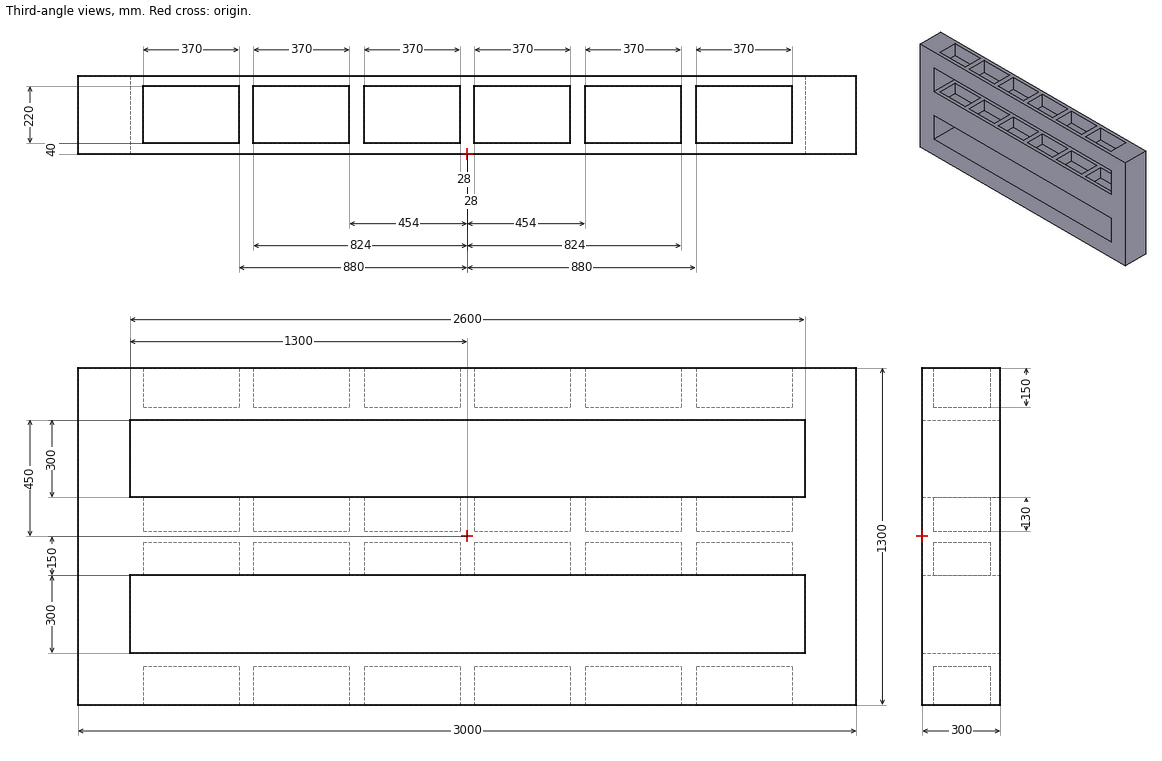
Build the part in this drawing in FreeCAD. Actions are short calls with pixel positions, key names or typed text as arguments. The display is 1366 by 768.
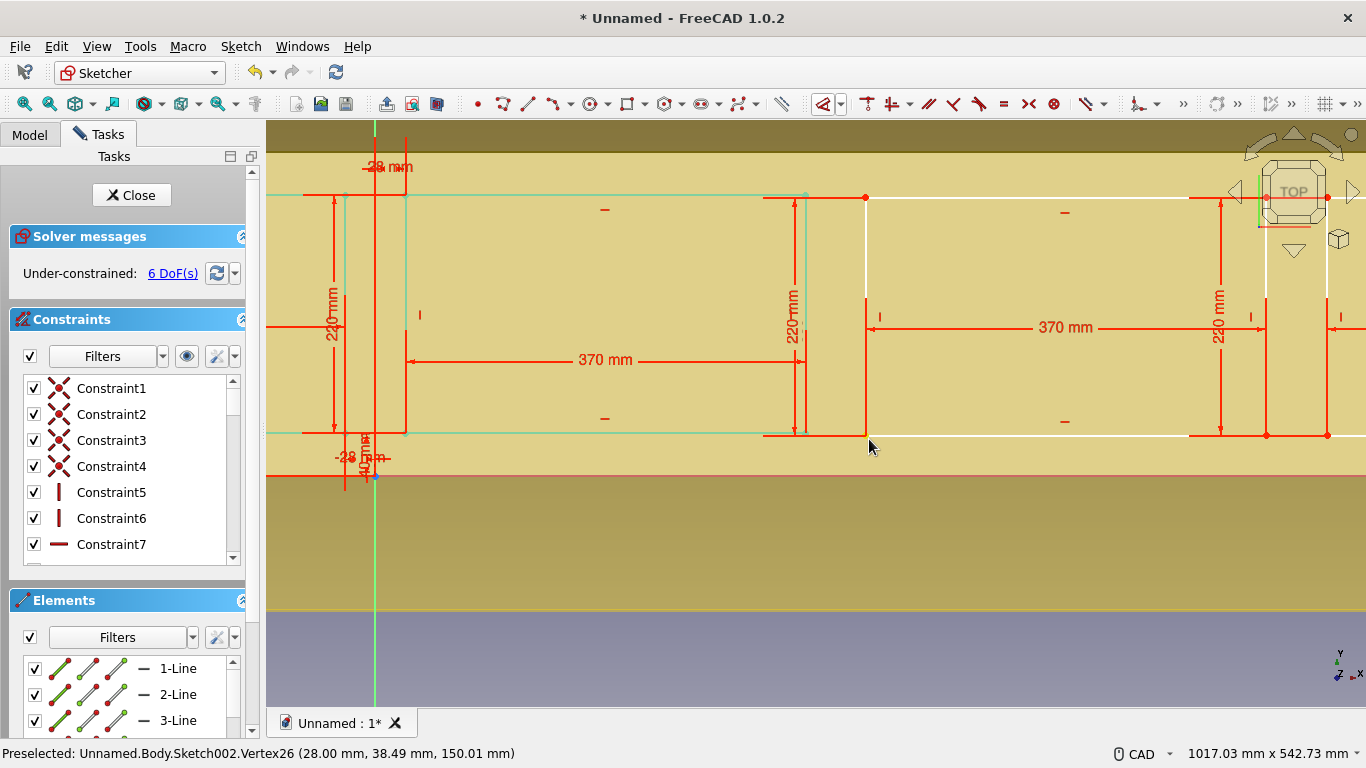
click(866, 436)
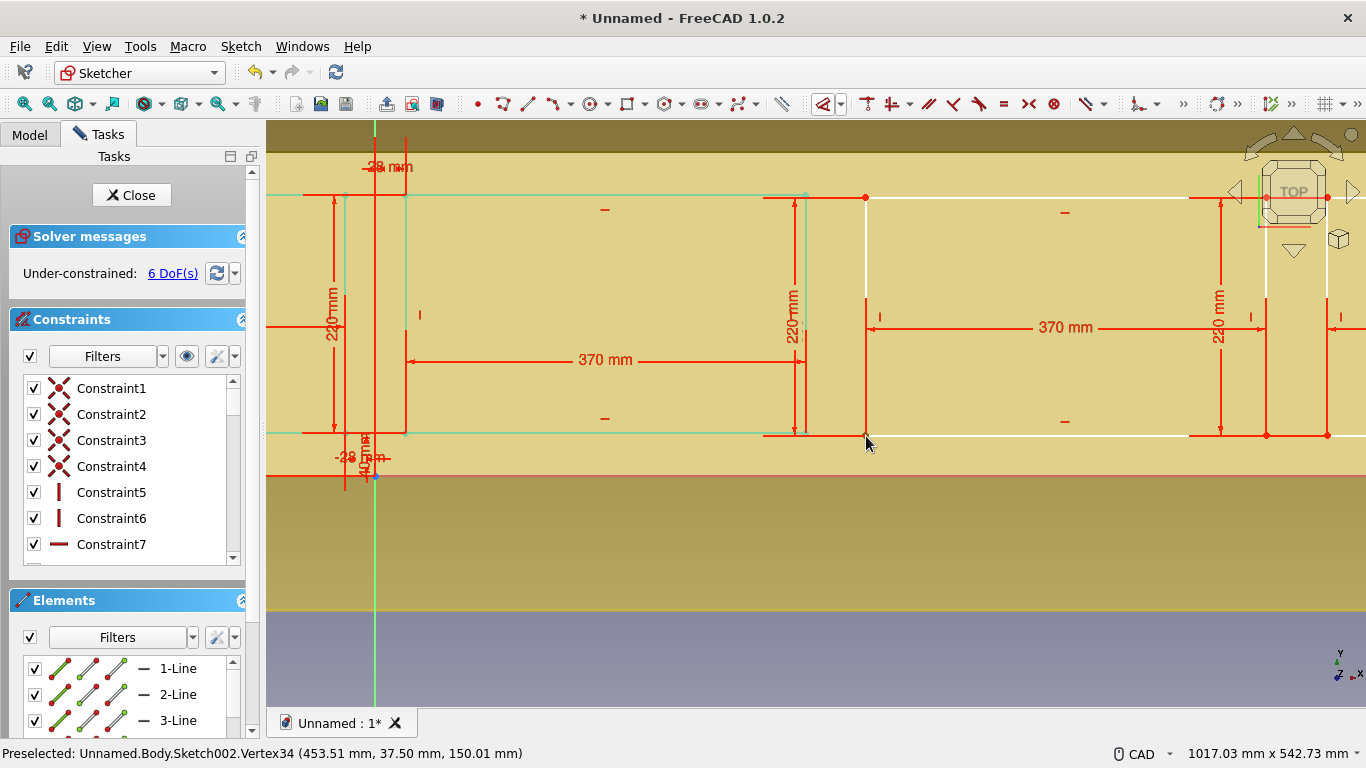
key(i)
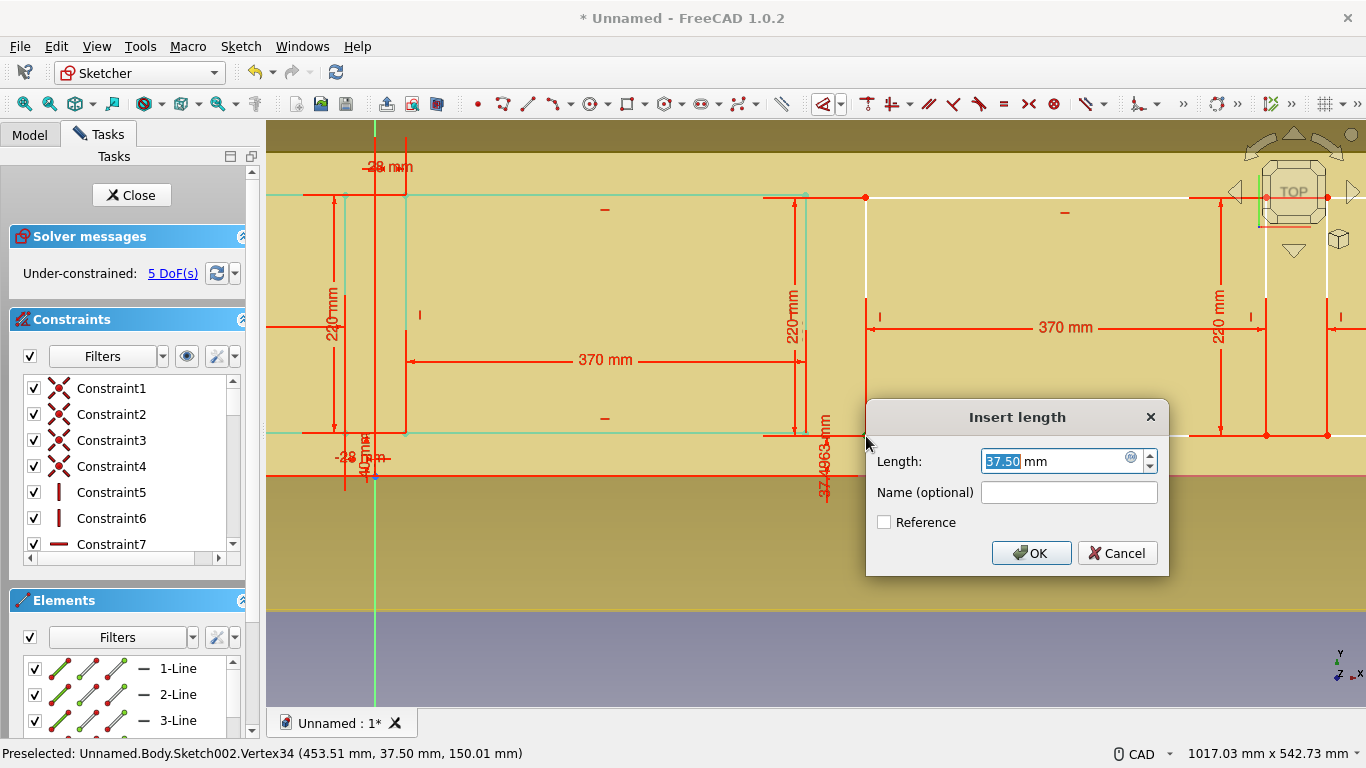
text(40)
key(Return)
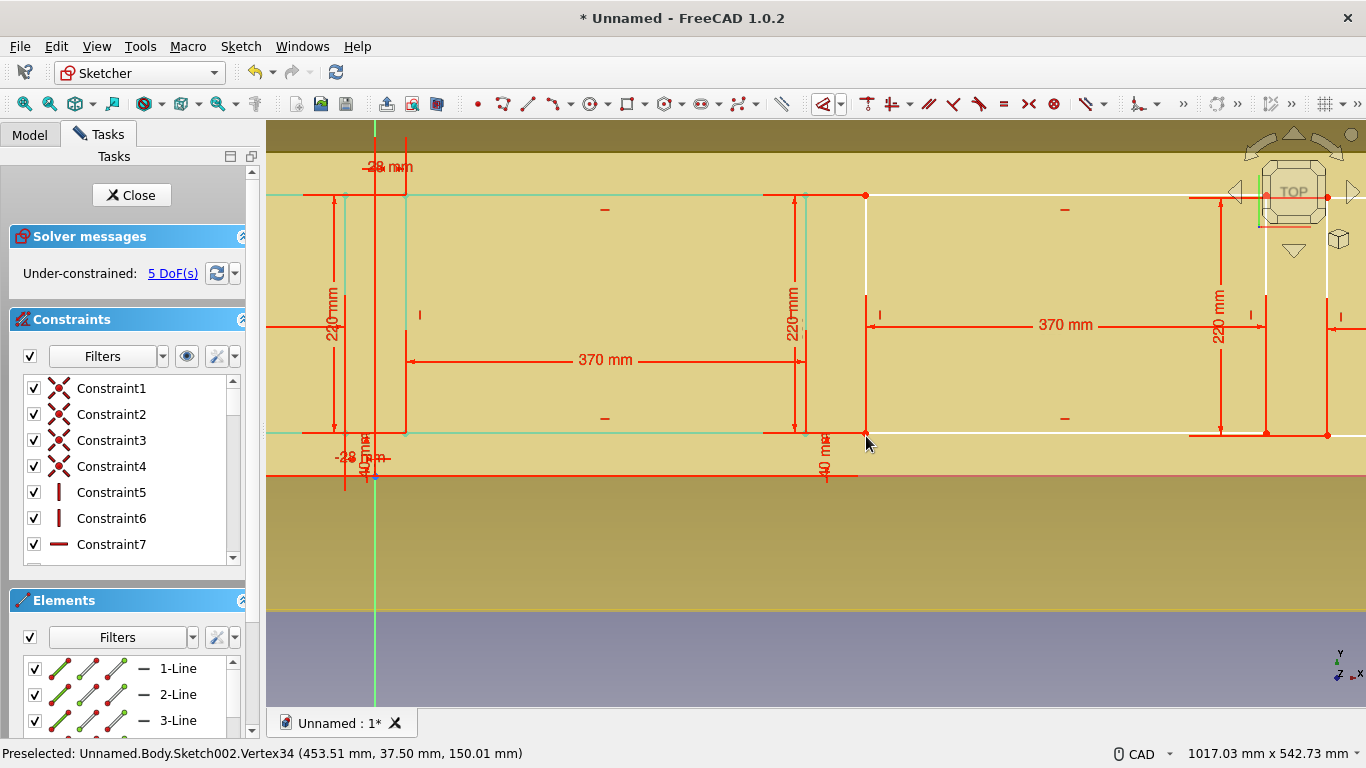
scroll(869, 439, down, 7)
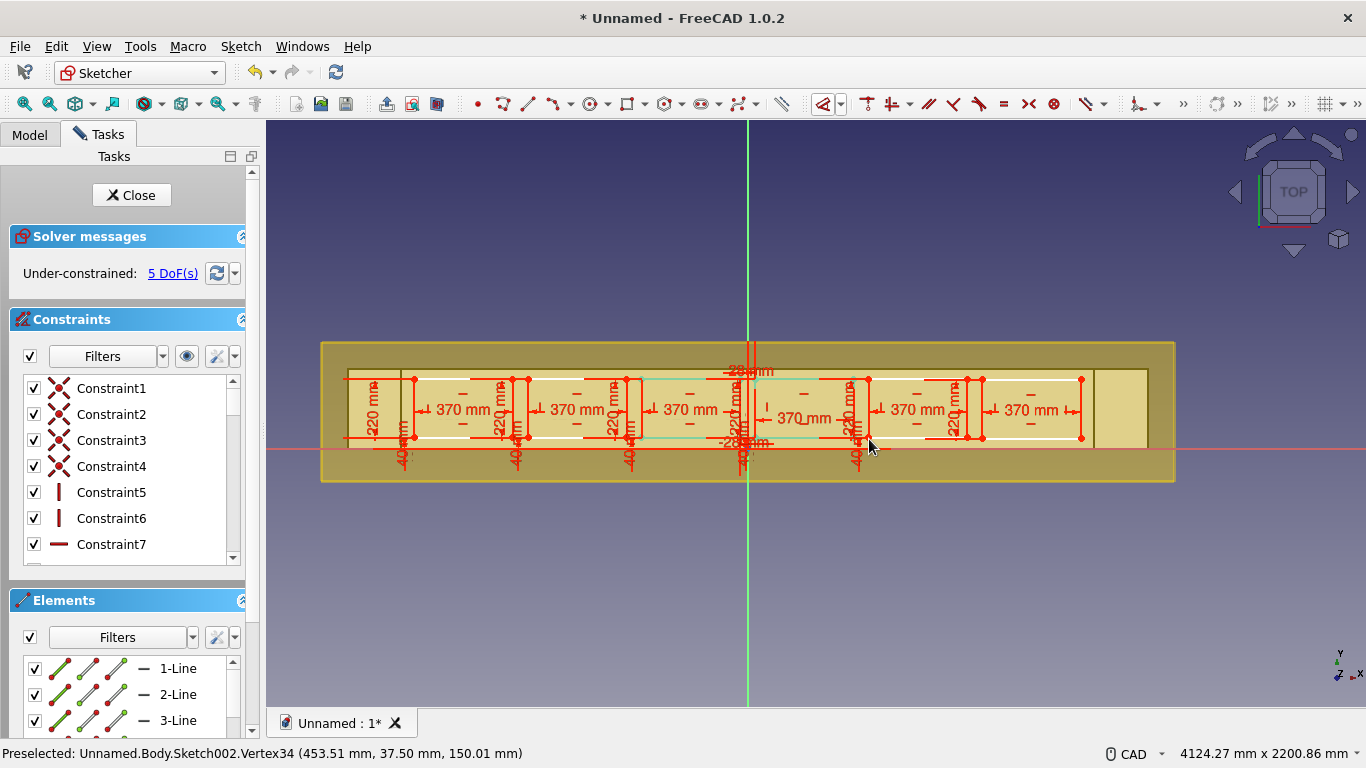
scroll(982, 439, up, 7)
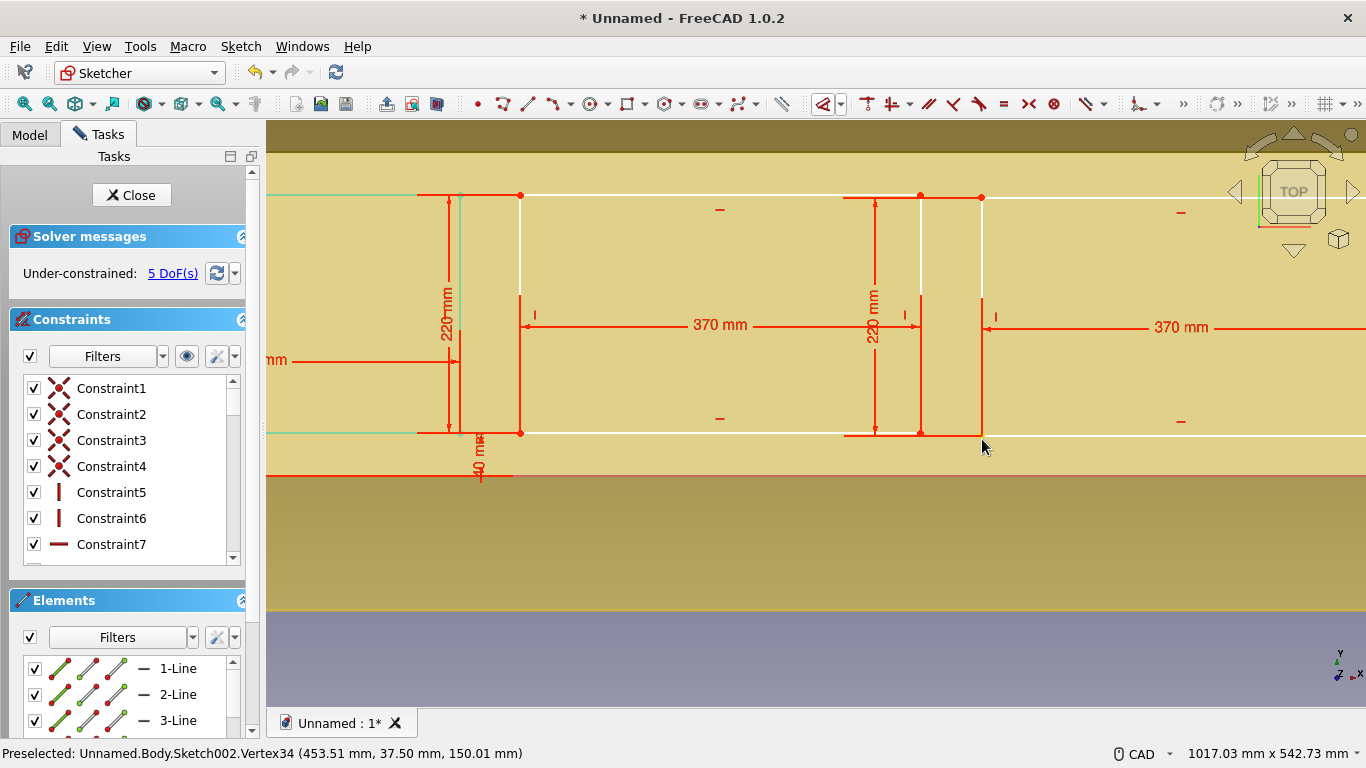
click(982, 436)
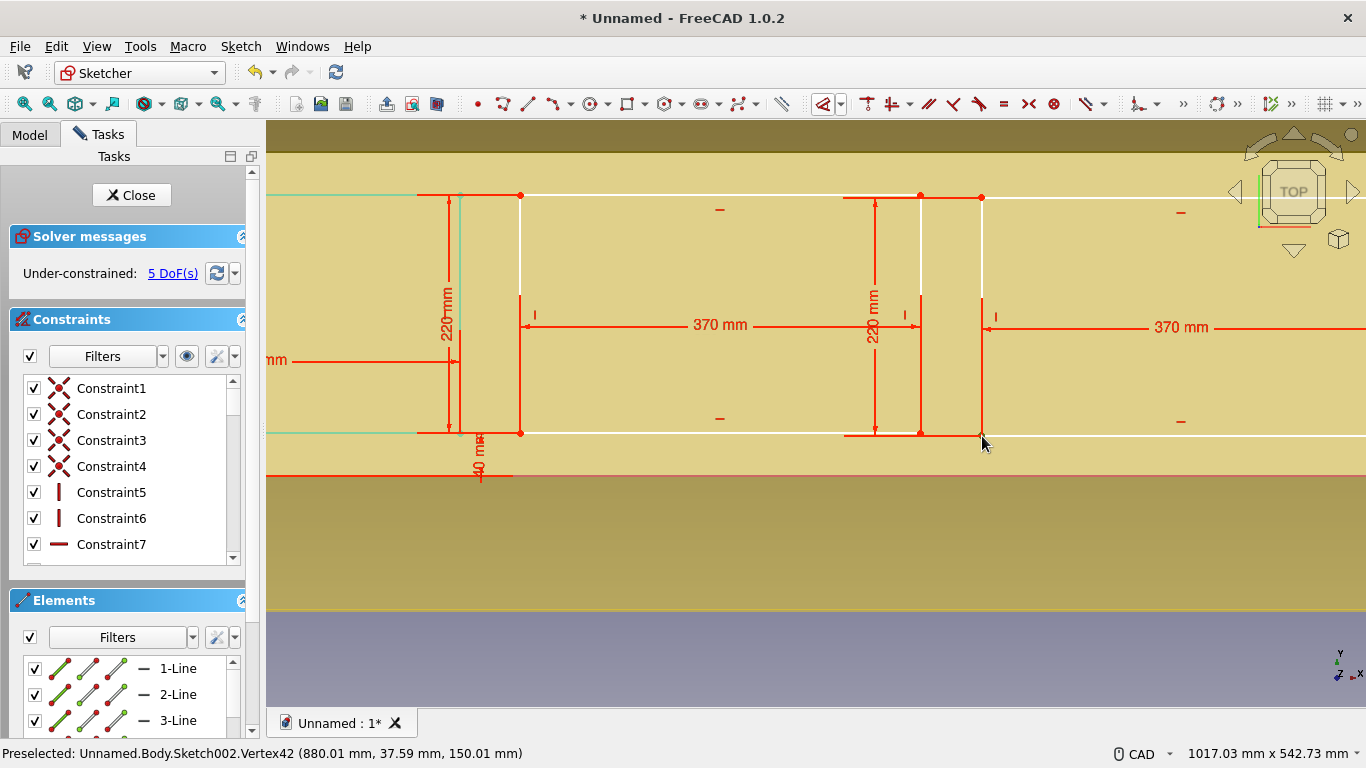
key(i)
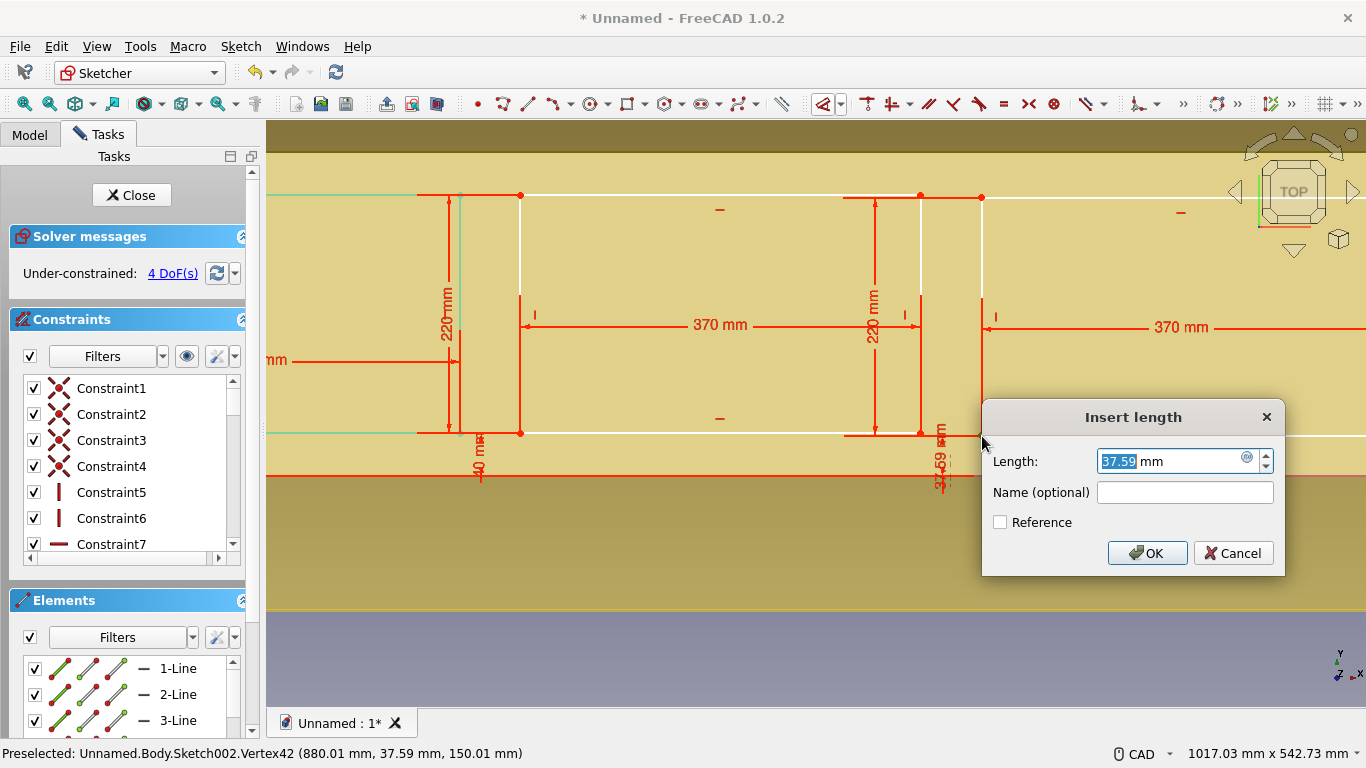
text(40)
key(Return)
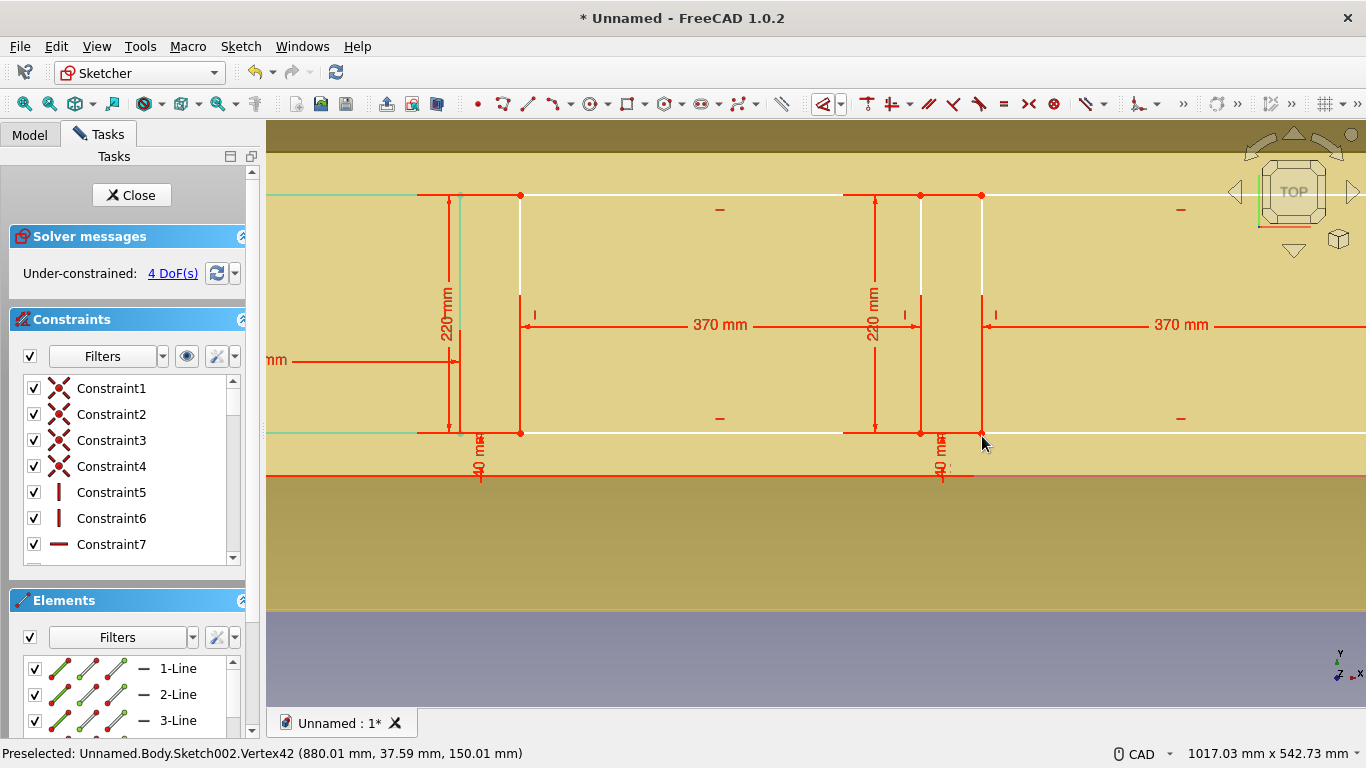
scroll(982, 439, down, 7)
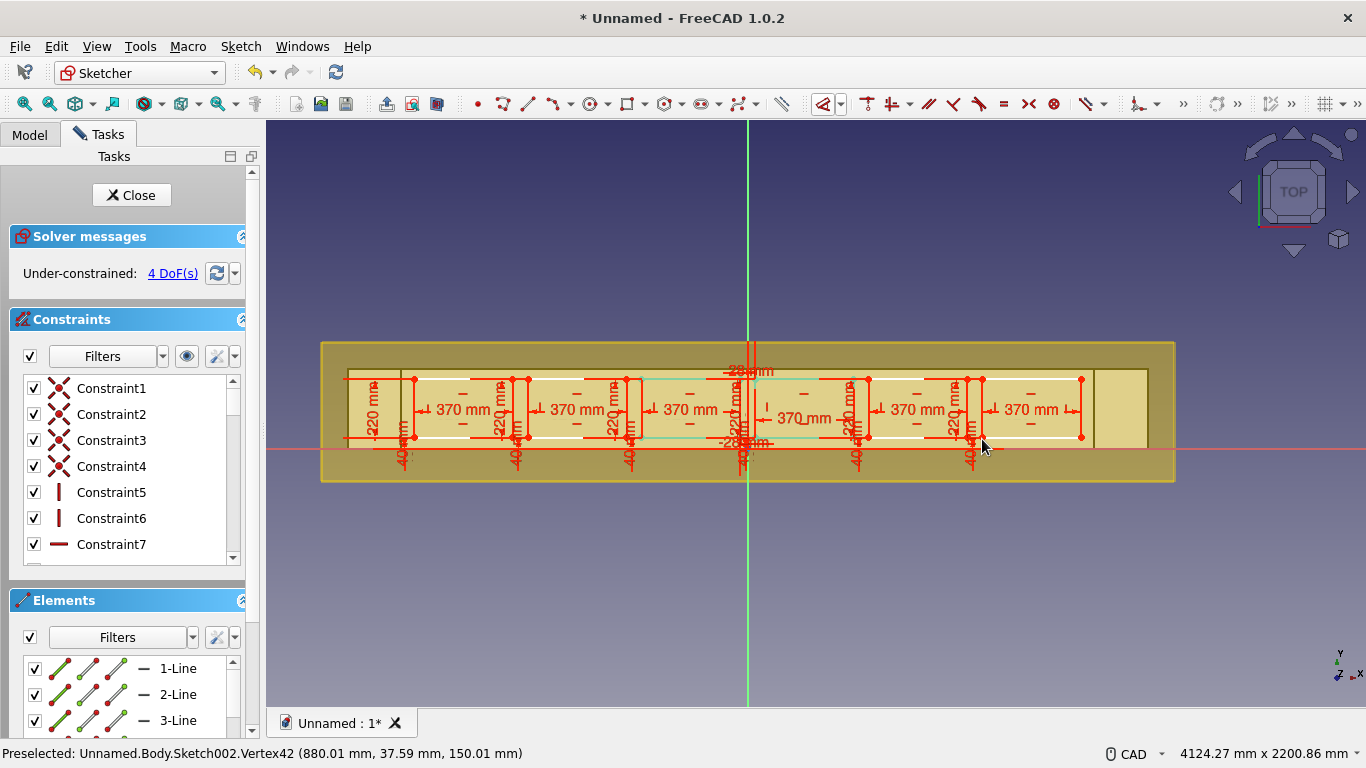
click(513, 438)